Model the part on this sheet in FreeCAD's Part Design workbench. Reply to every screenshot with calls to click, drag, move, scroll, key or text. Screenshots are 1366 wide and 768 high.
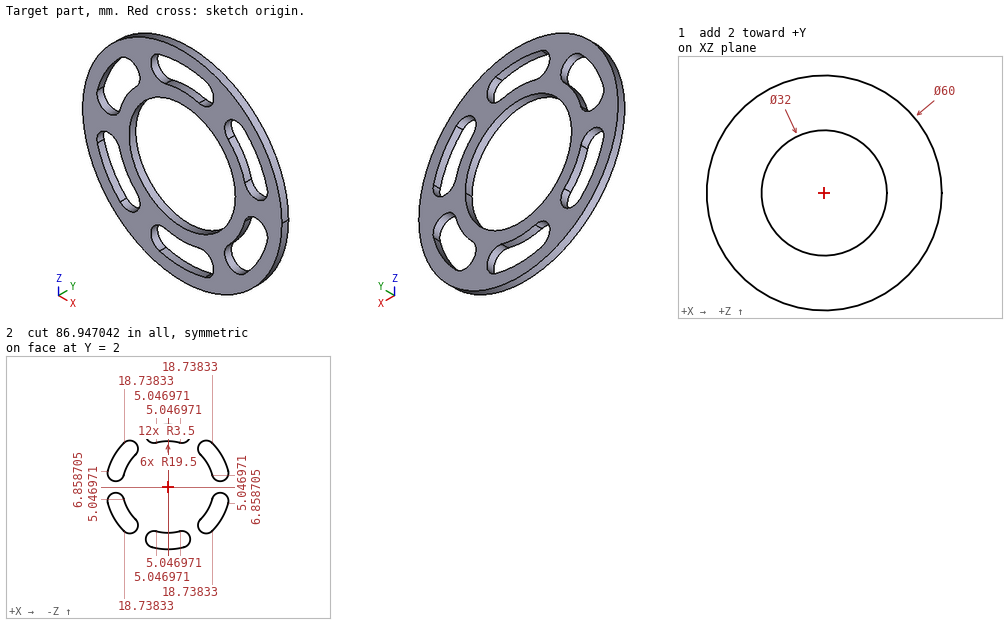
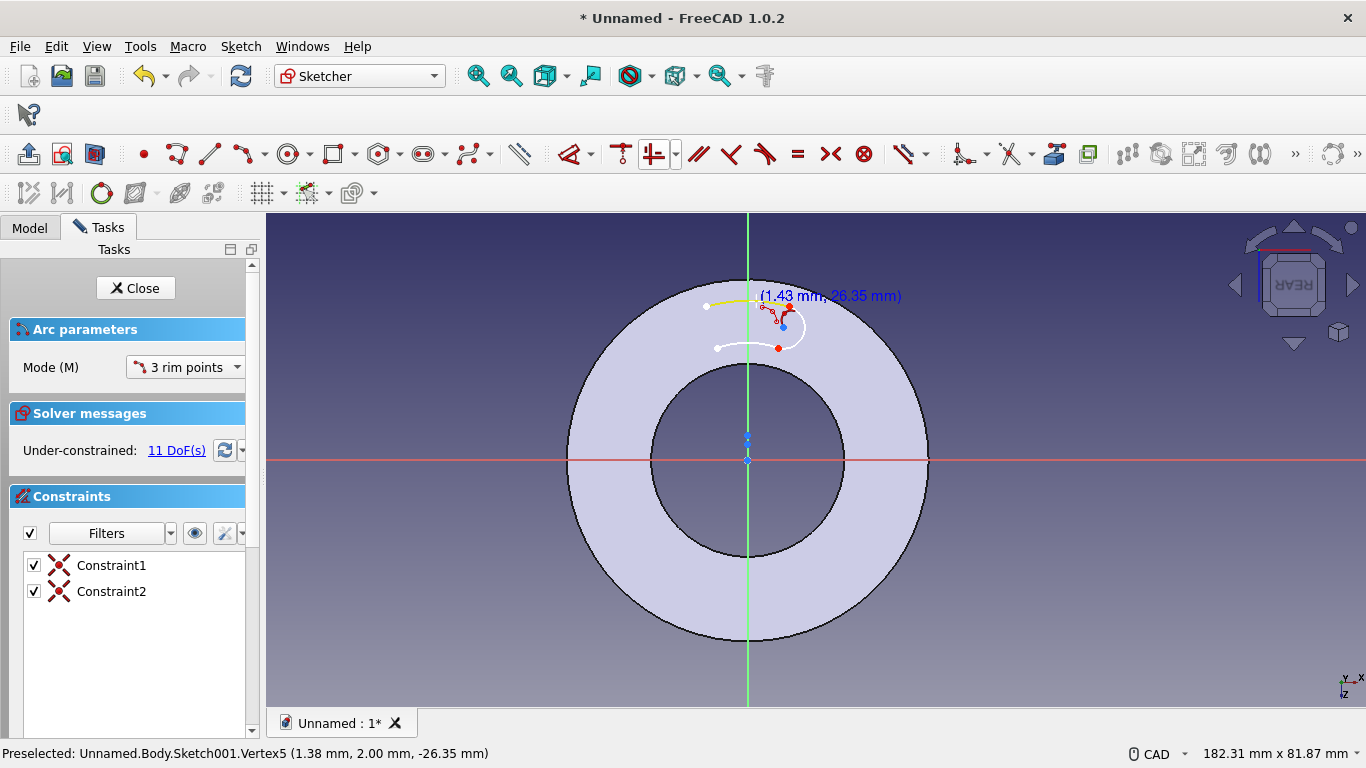
click(706, 307)
click(717, 348)
click(691, 332)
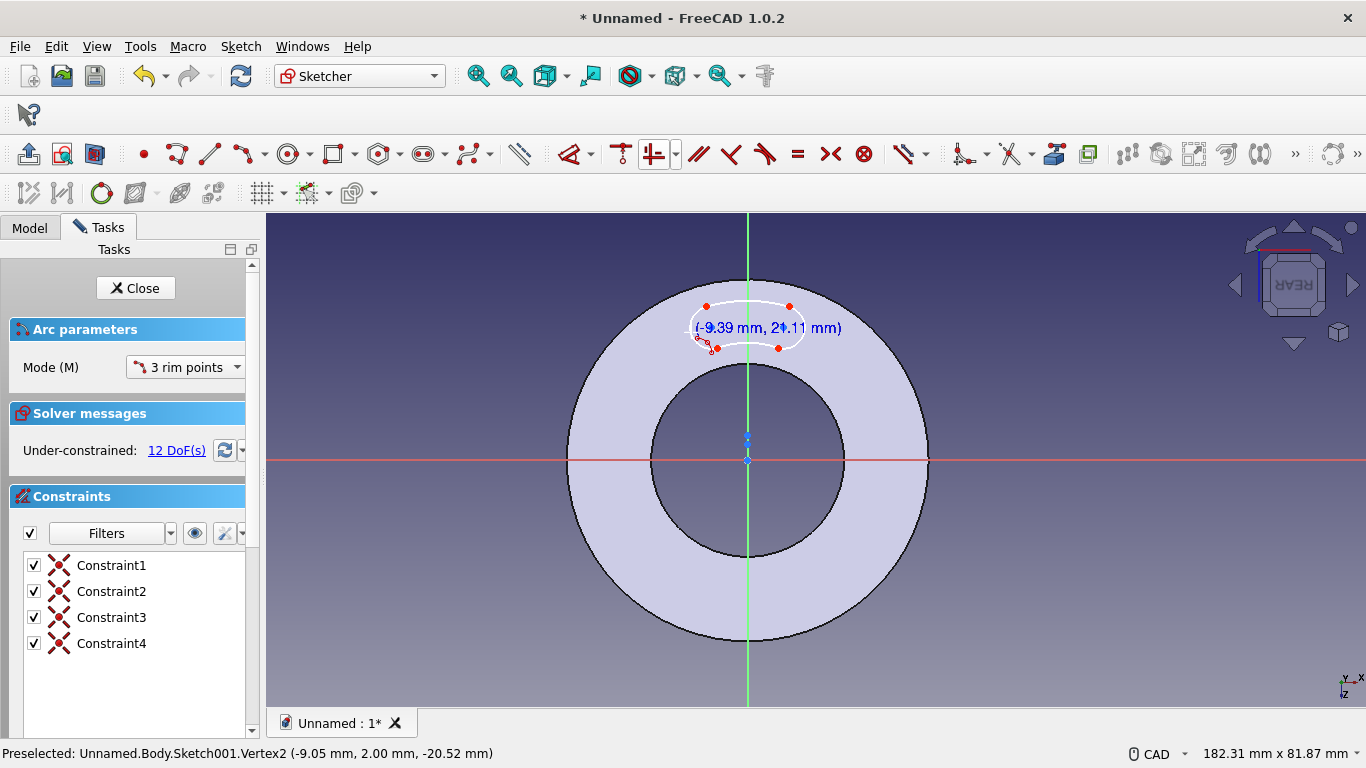
click(831, 377)
click(861, 430)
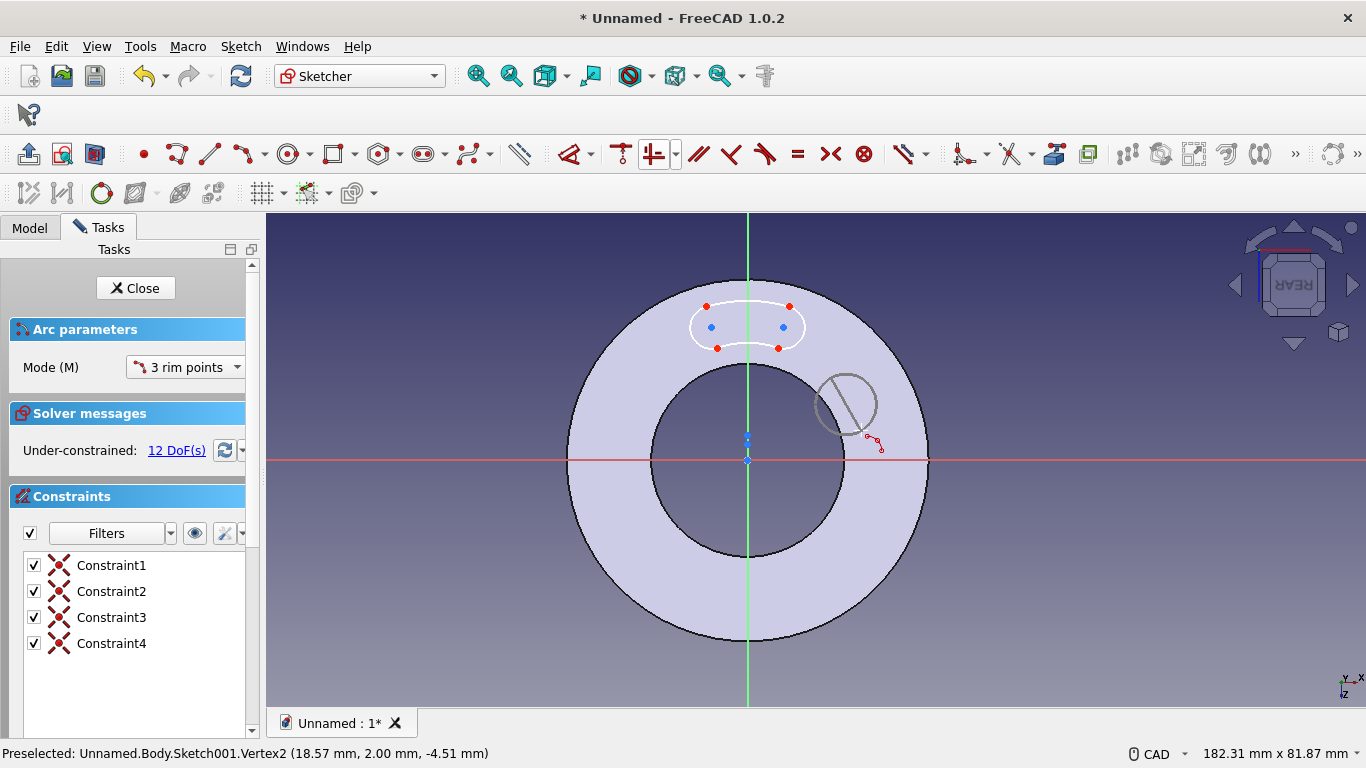
scroll(850, 402, up, 7)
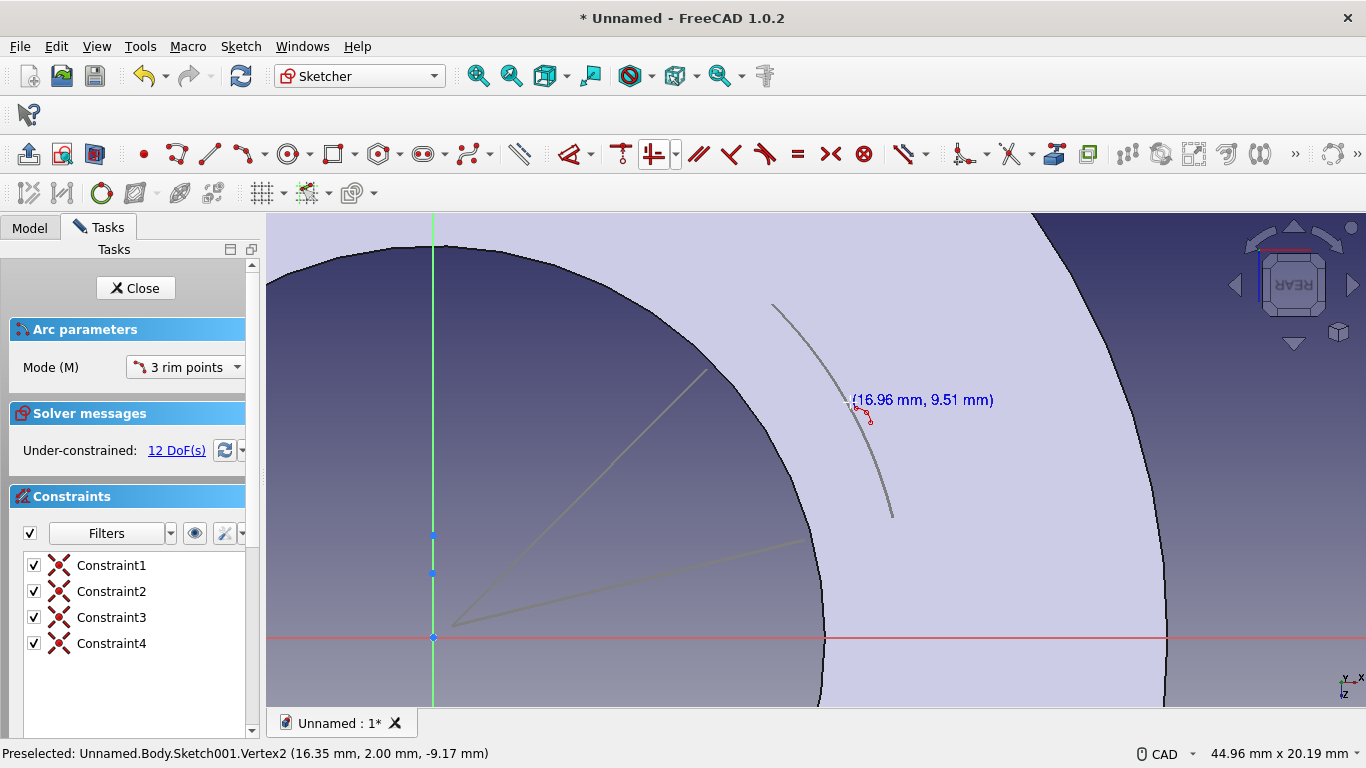
click(847, 399)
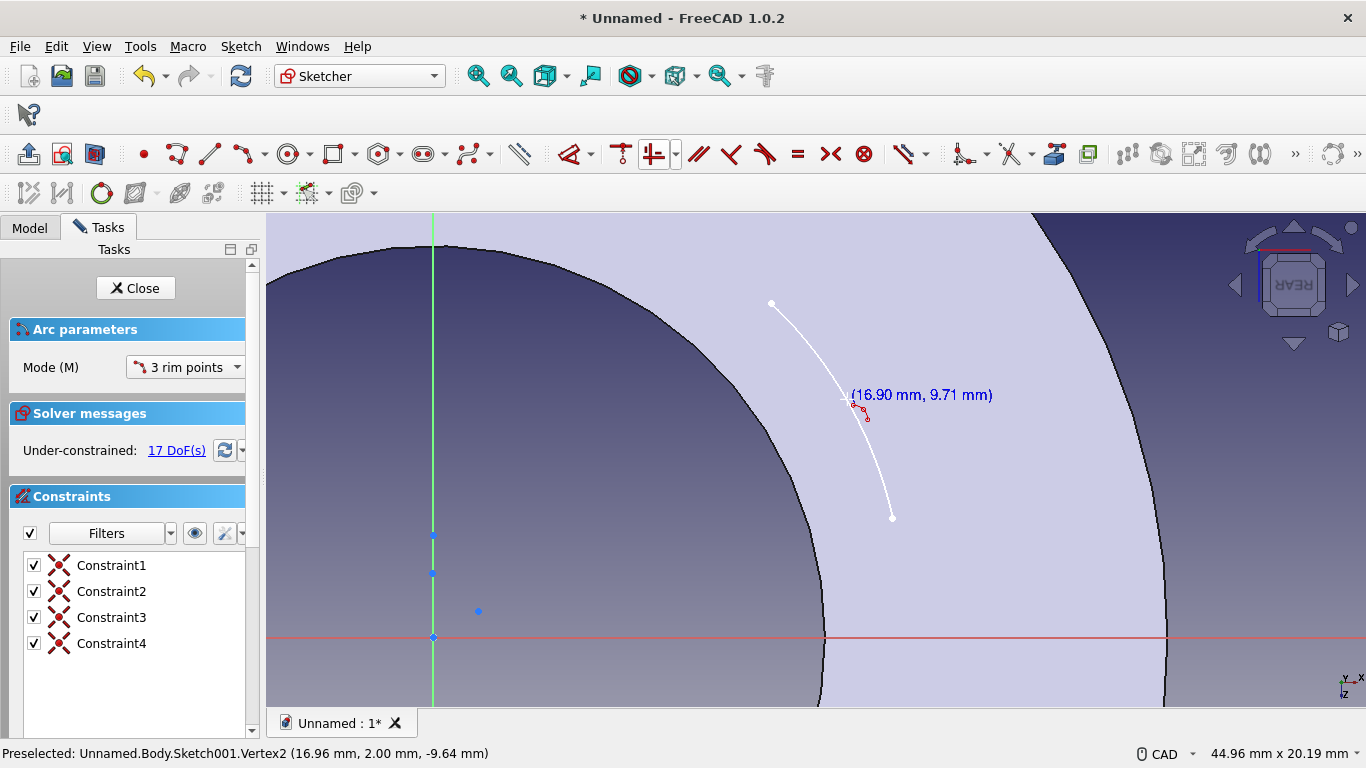
scroll(850, 402, down, 7)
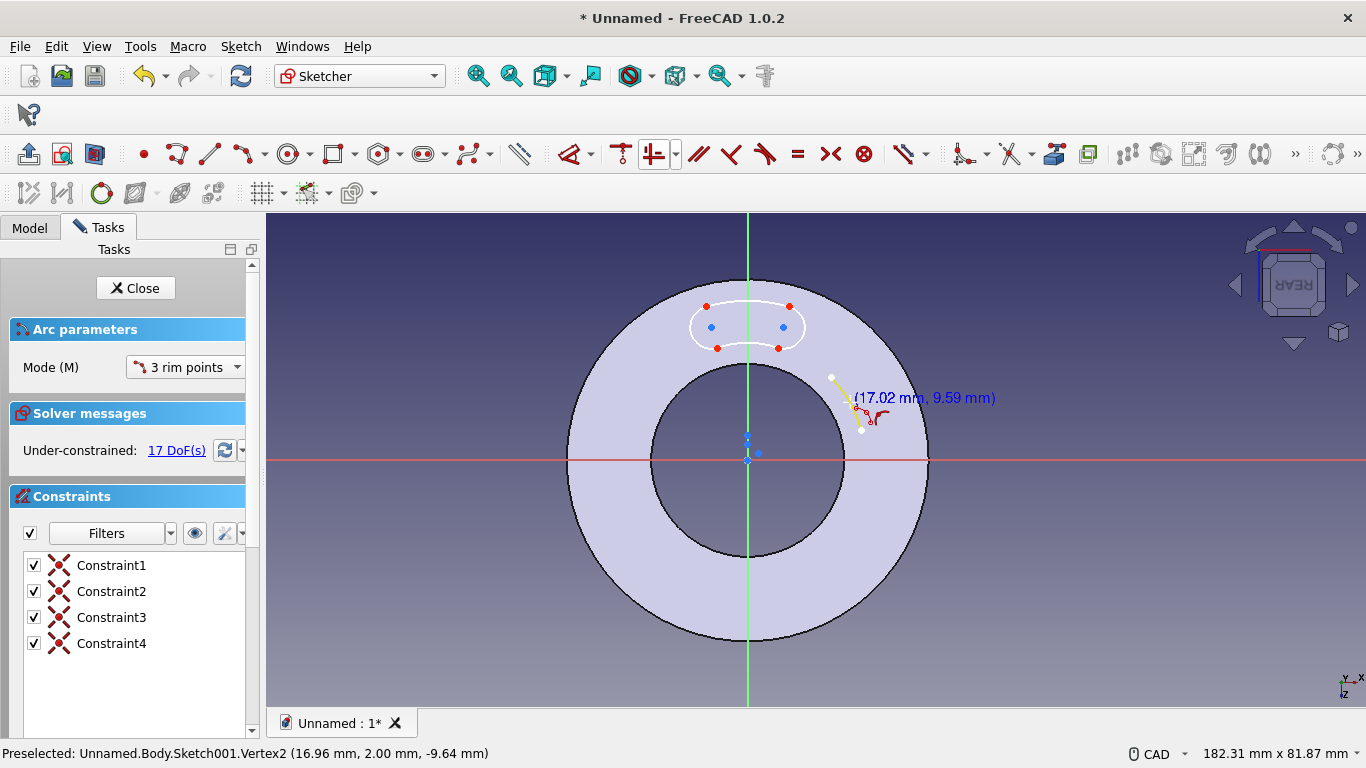
click(861, 431)
click(902, 419)
click(893, 442)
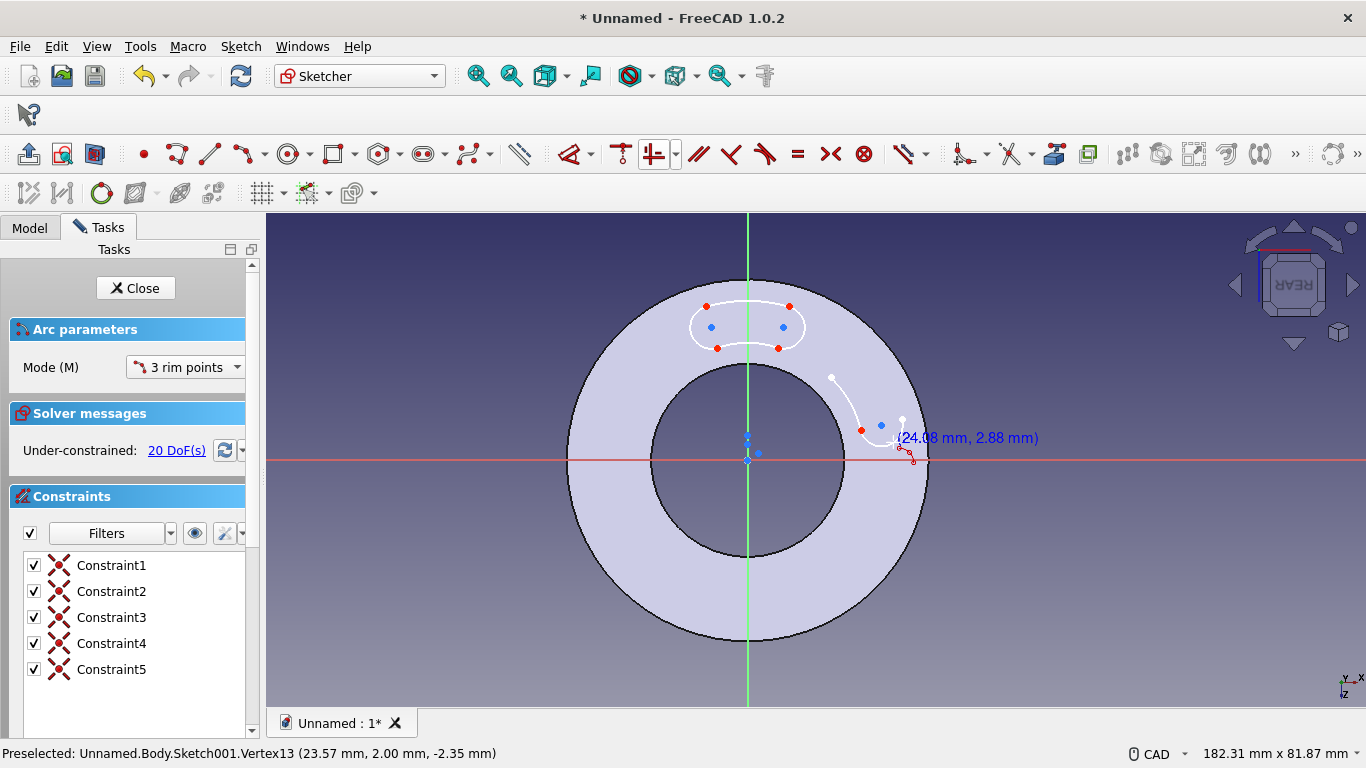
click(902, 420)
click(861, 347)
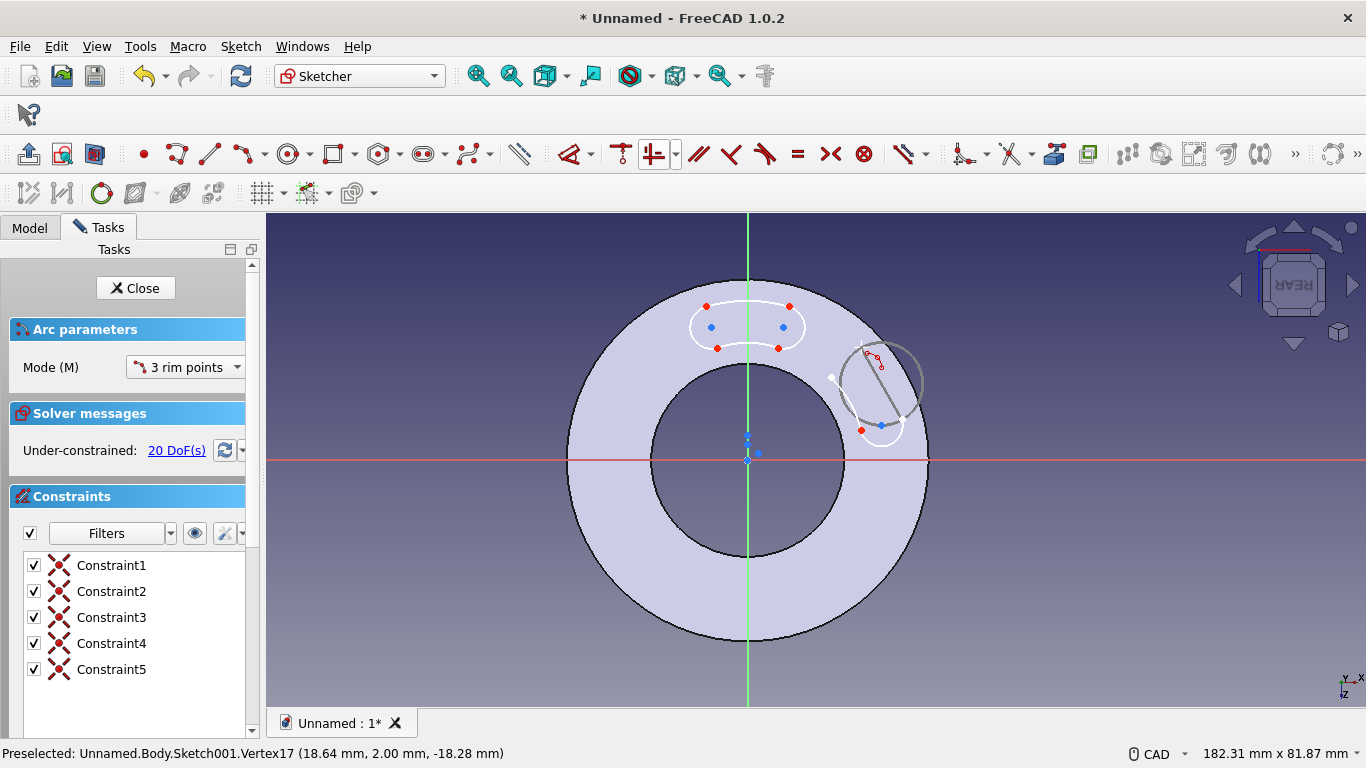
scroll(886, 380, up, 6)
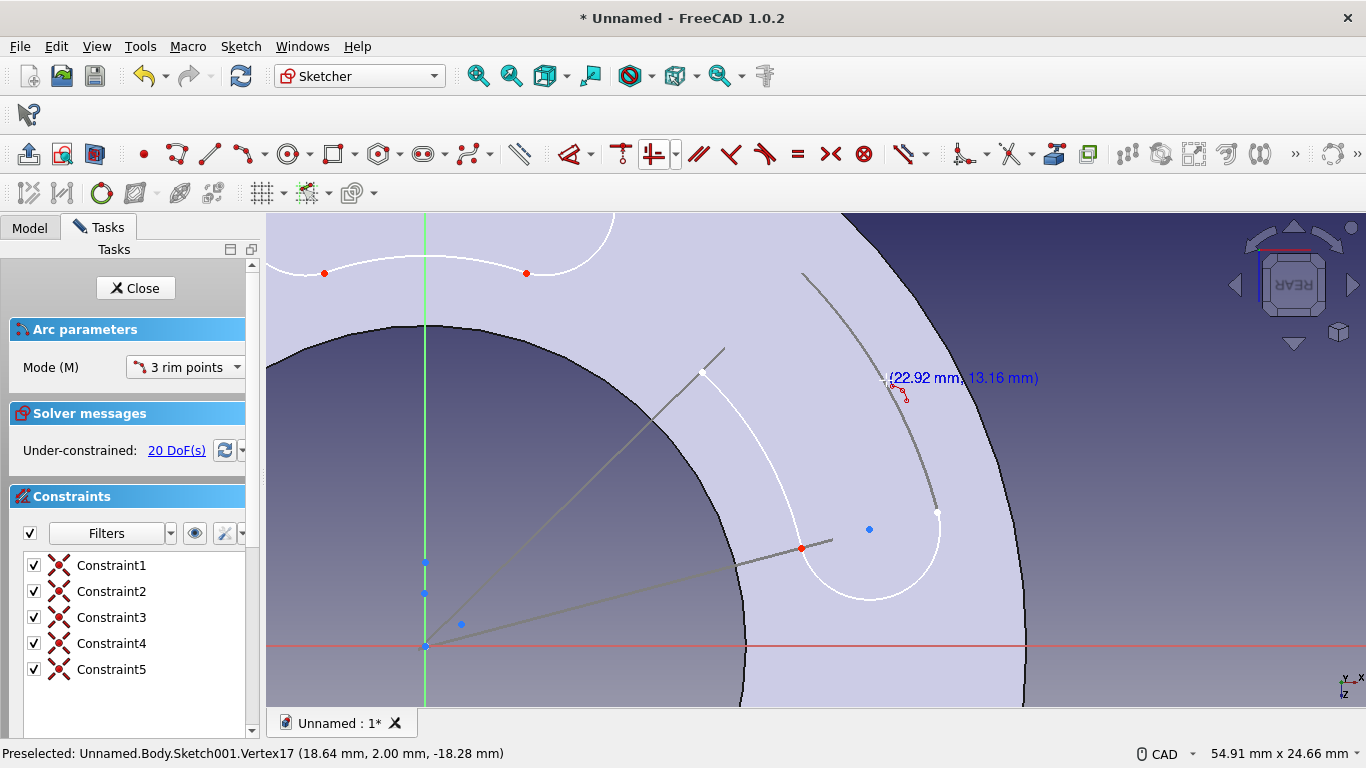
click(885, 381)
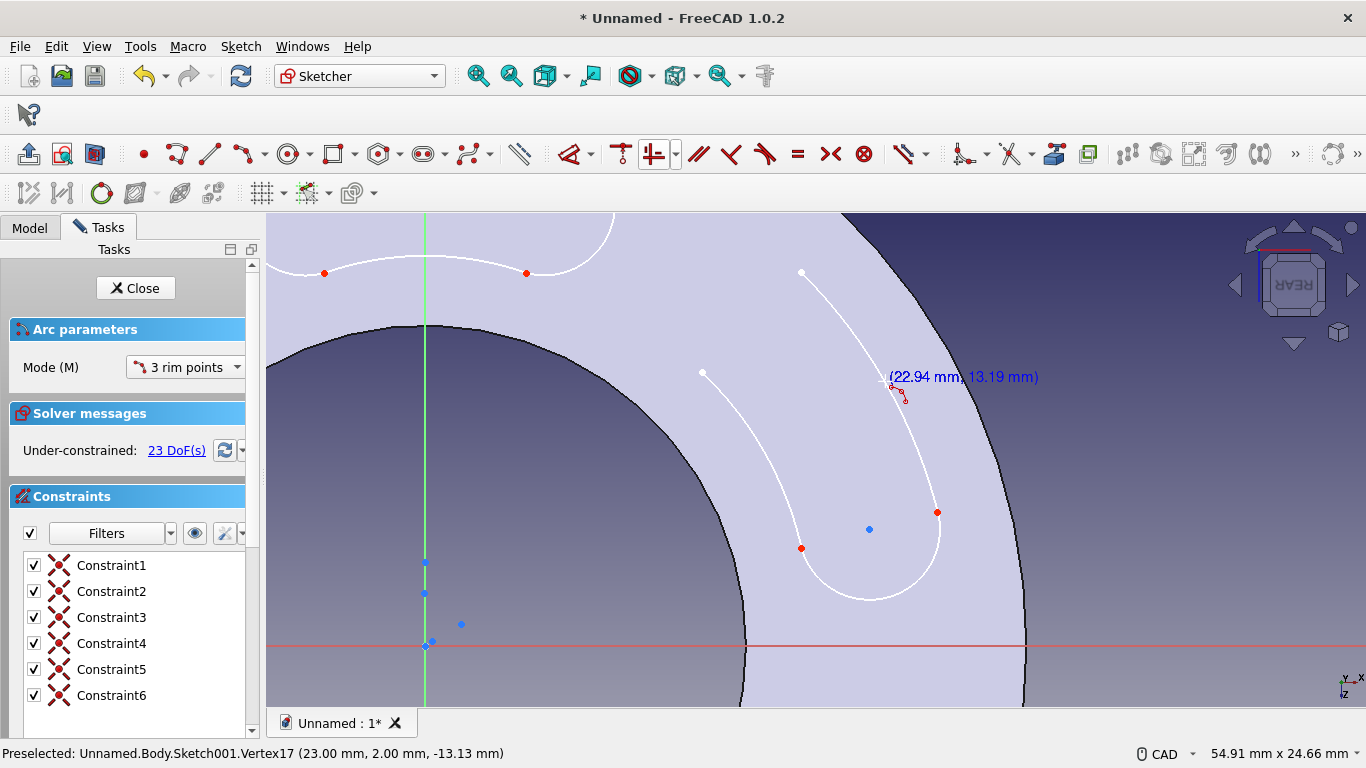
scroll(886, 380, down, 6)